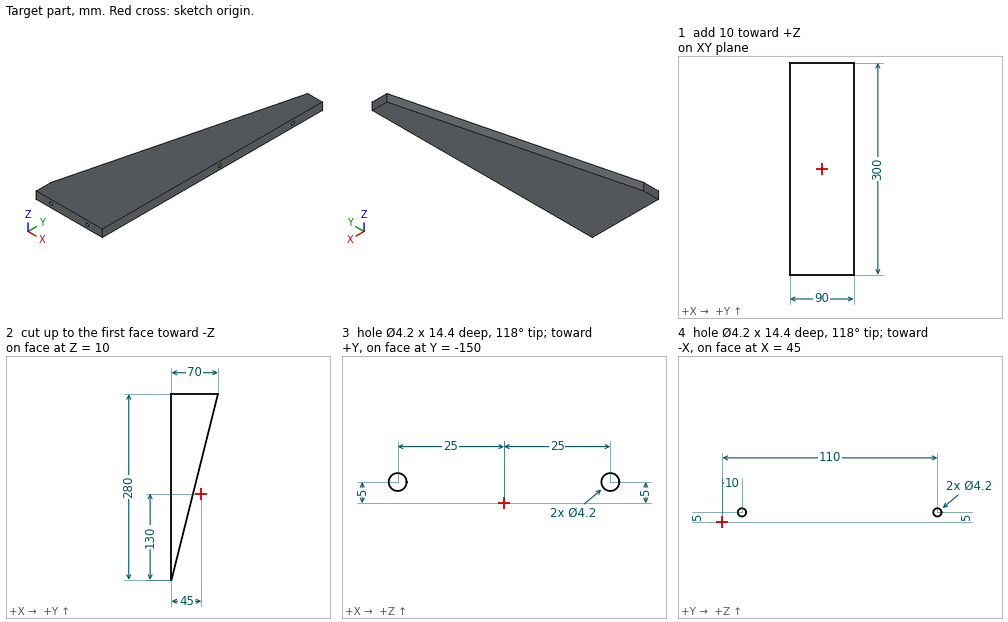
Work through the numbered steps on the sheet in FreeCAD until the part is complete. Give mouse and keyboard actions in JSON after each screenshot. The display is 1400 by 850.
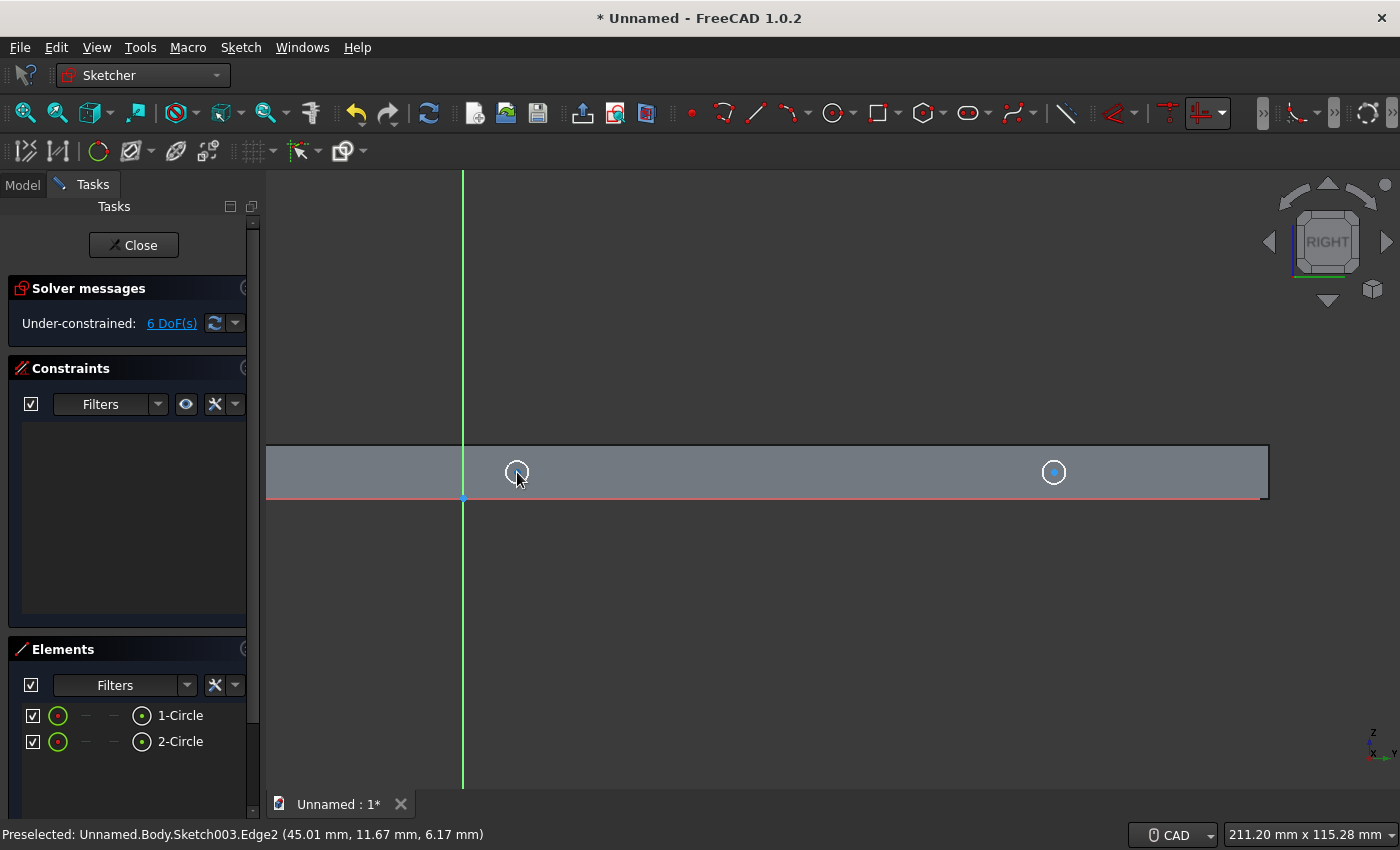
{"action": "left_click", "coordinate": [1062, 464]}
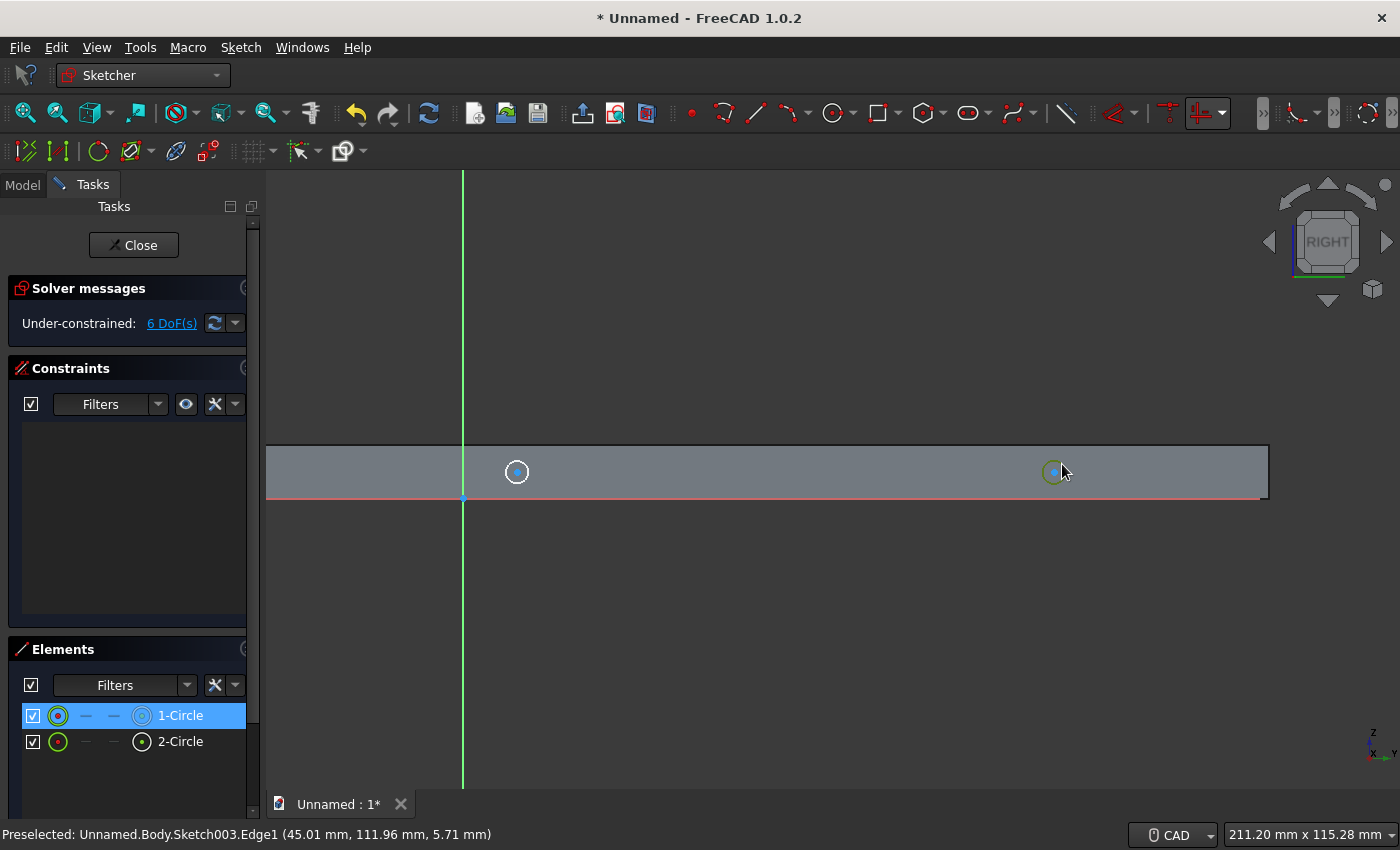
{"action": "scroll", "coordinate": [525, 464], "scroll_direction": "up", "scroll_amount": 2}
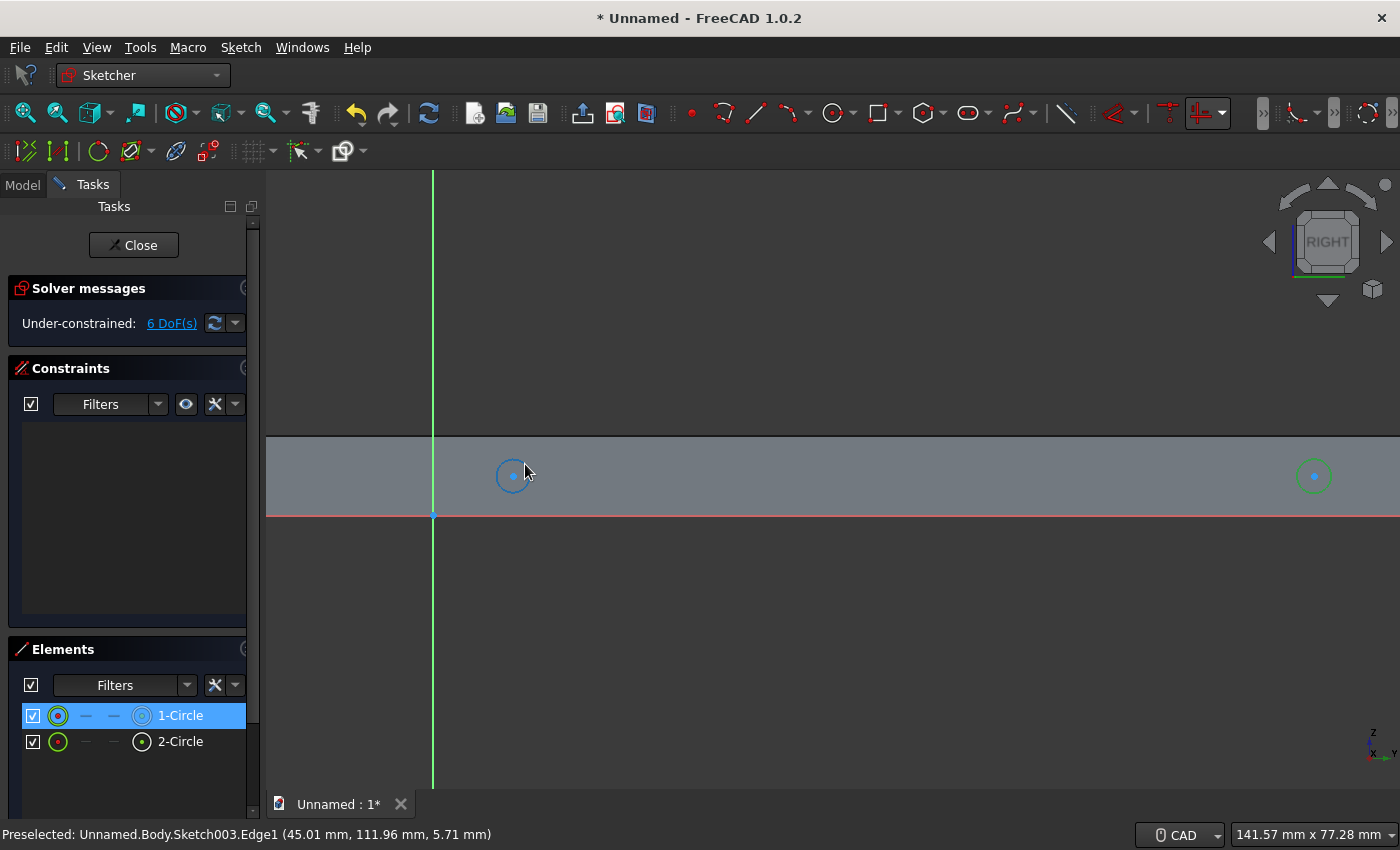
{"action": "left_click", "coordinate": [525, 464]}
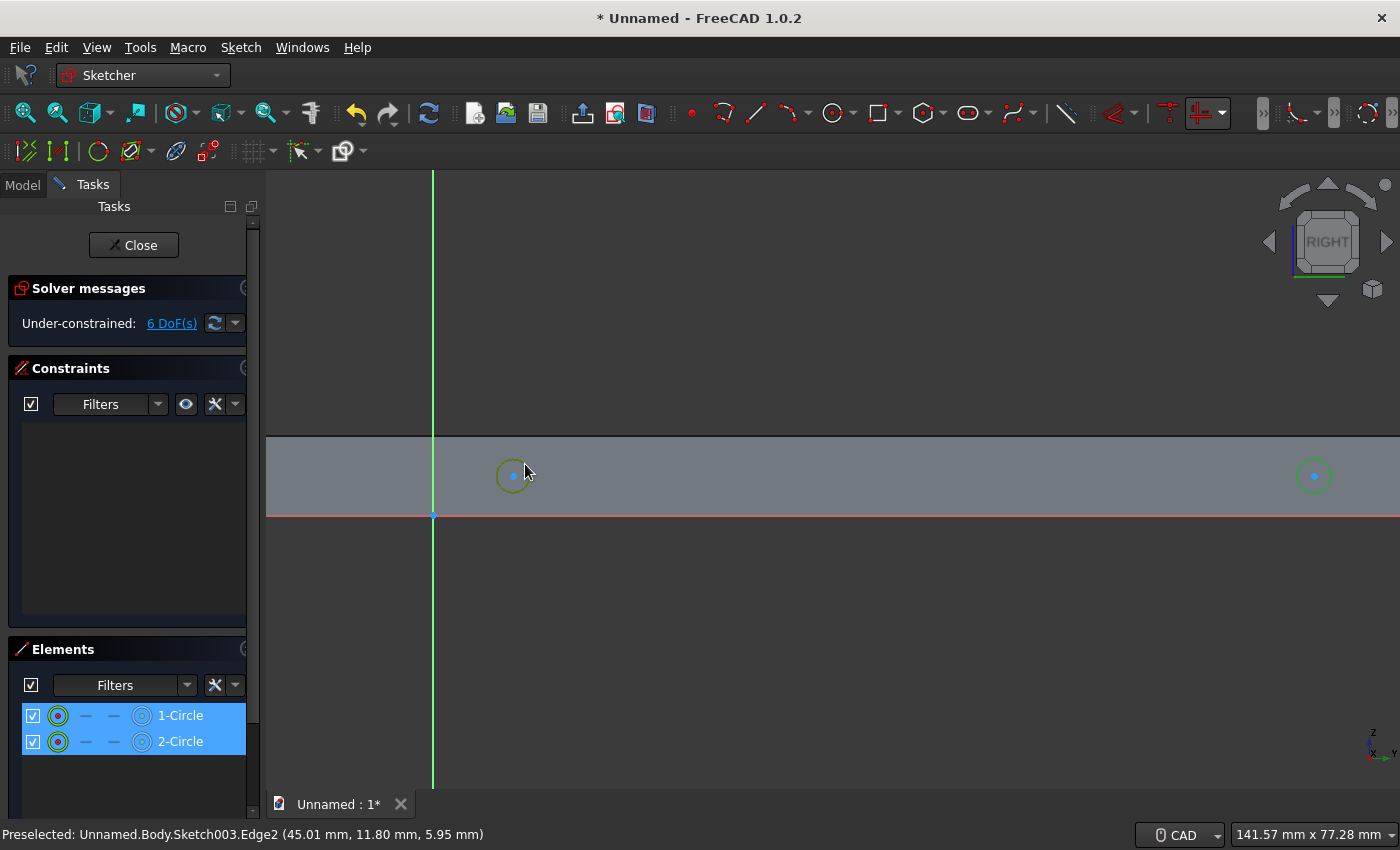
{"action": "key", "text": "e"}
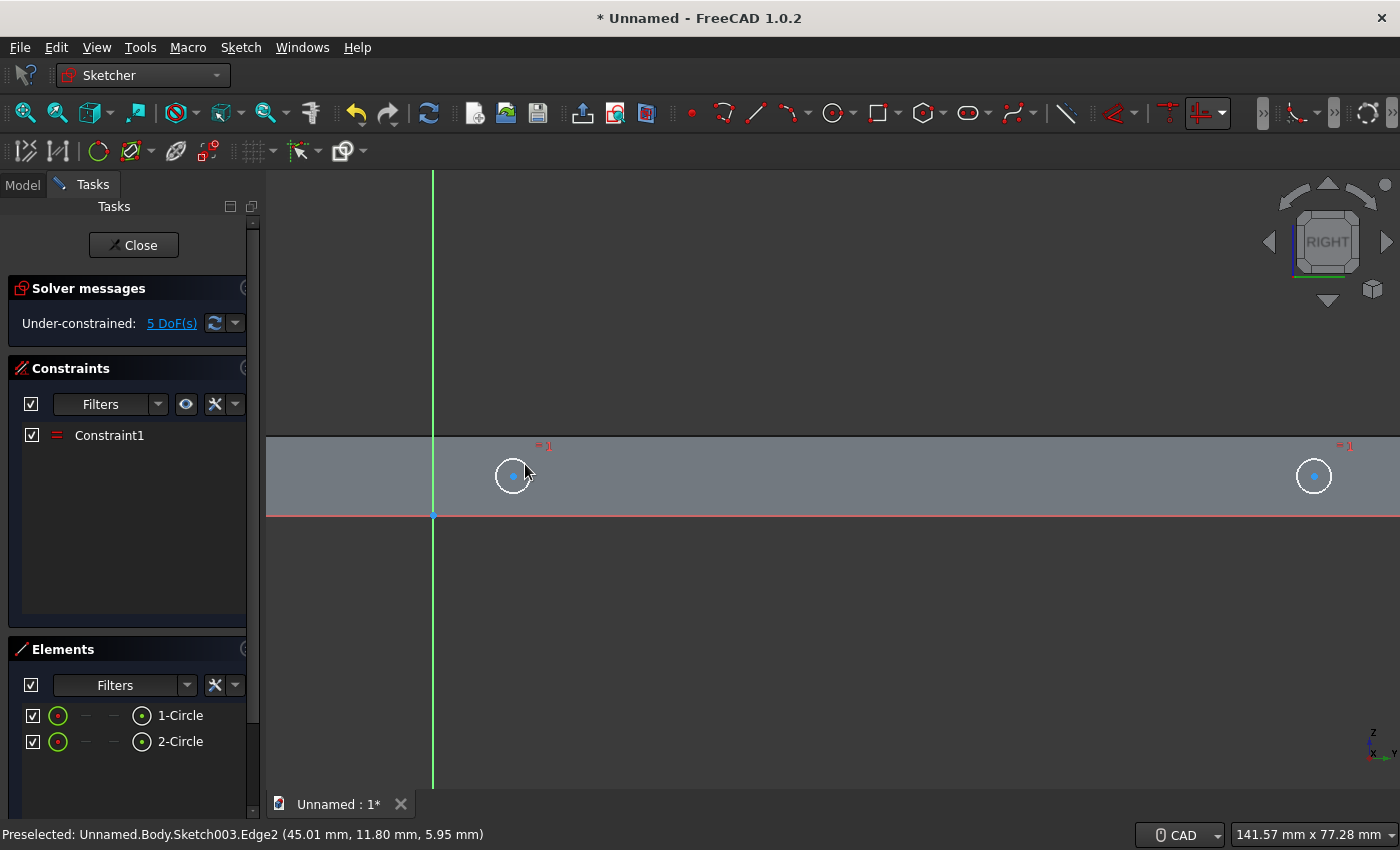
{"action": "key", "text": "d"}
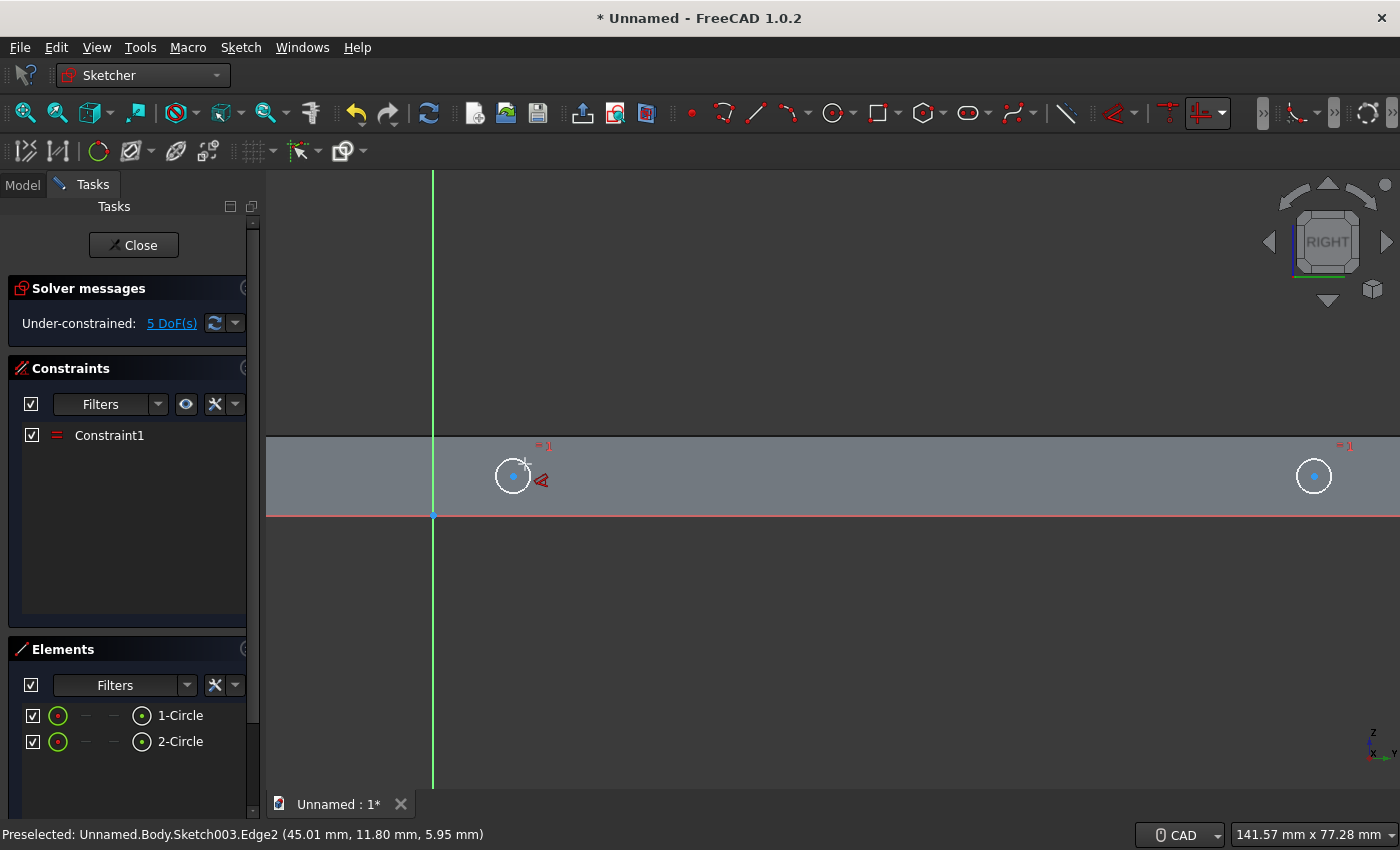
{"action": "scroll", "coordinate": [525, 464], "scroll_direction": "down", "scroll_amount": 2}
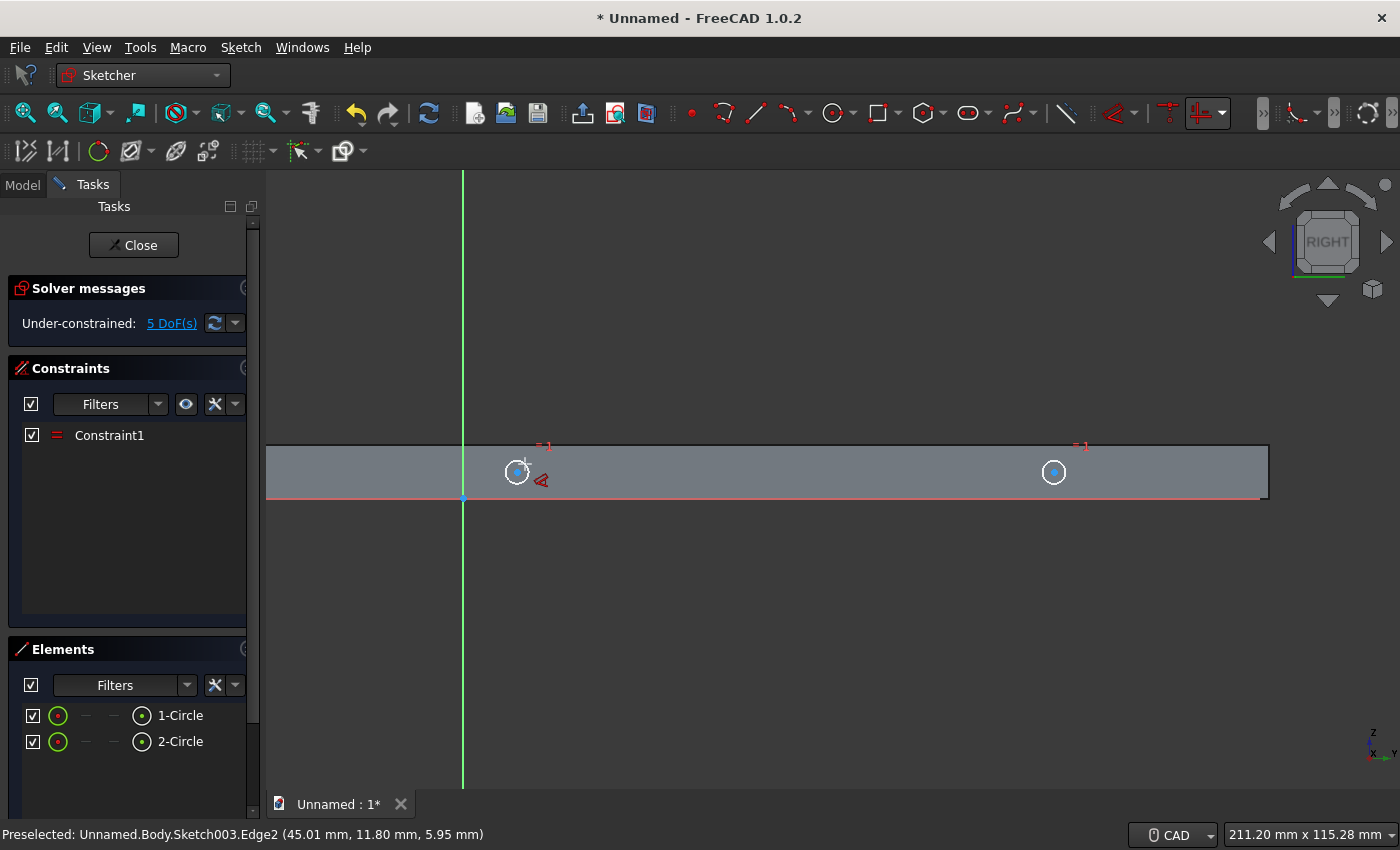
{"action": "scroll", "coordinate": [1062, 464], "scroll_direction": "up", "scroll_amount": 3}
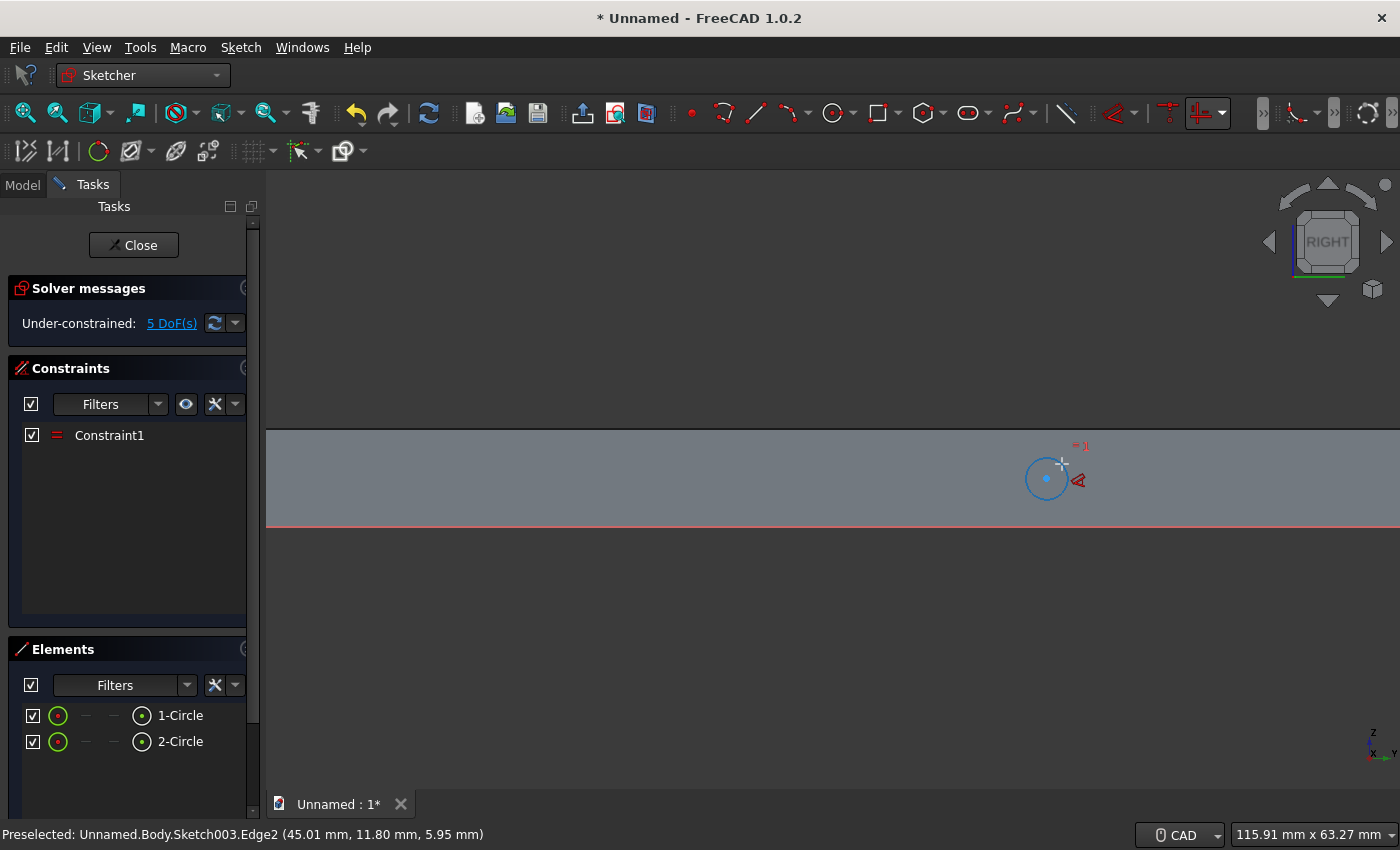
{"action": "left_click", "coordinate": [1062, 464]}
{"action": "left_click", "coordinate": [1085, 442]}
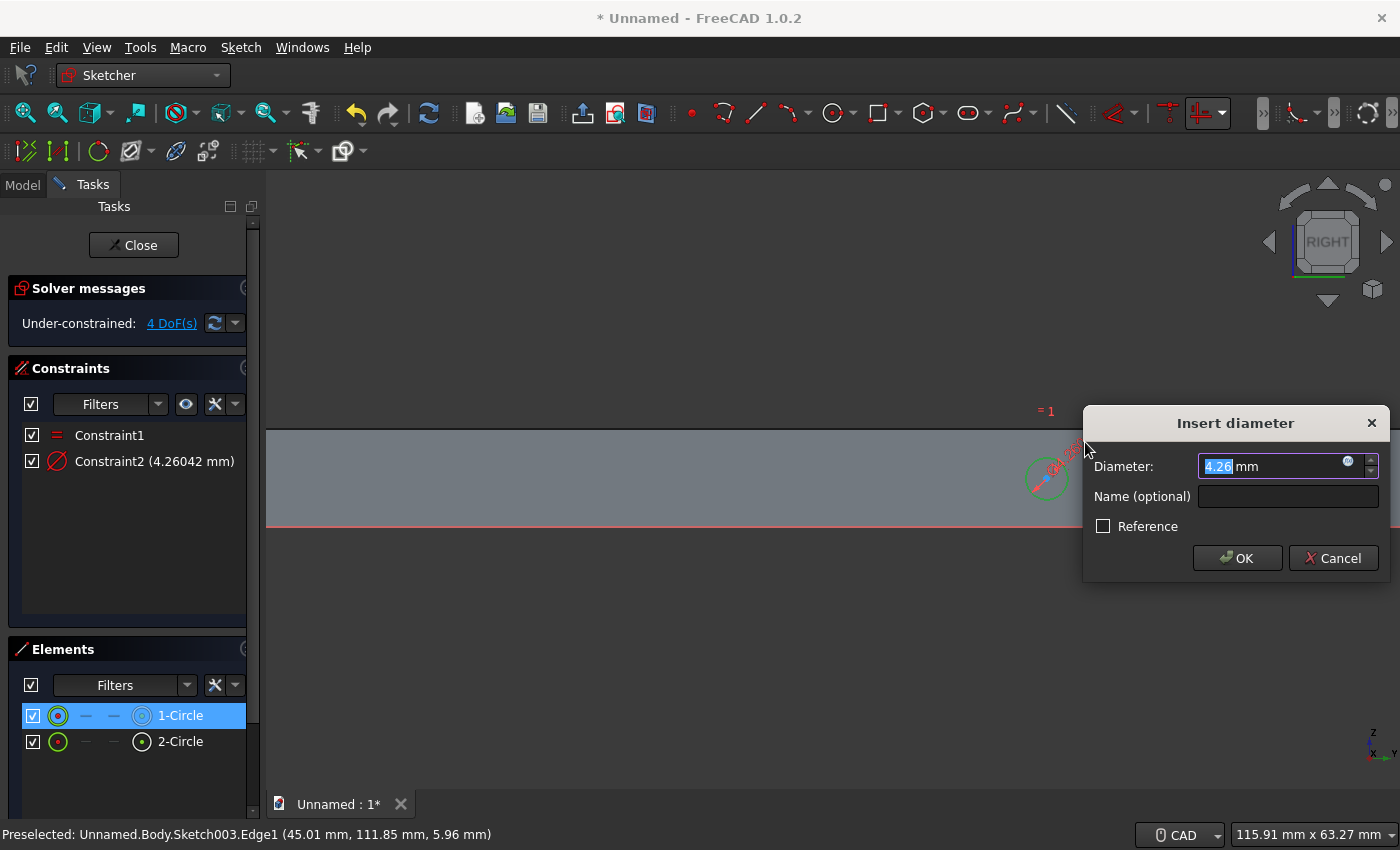
{"action": "type", "text": "4.2"}
{"action": "key", "text": "Return"}